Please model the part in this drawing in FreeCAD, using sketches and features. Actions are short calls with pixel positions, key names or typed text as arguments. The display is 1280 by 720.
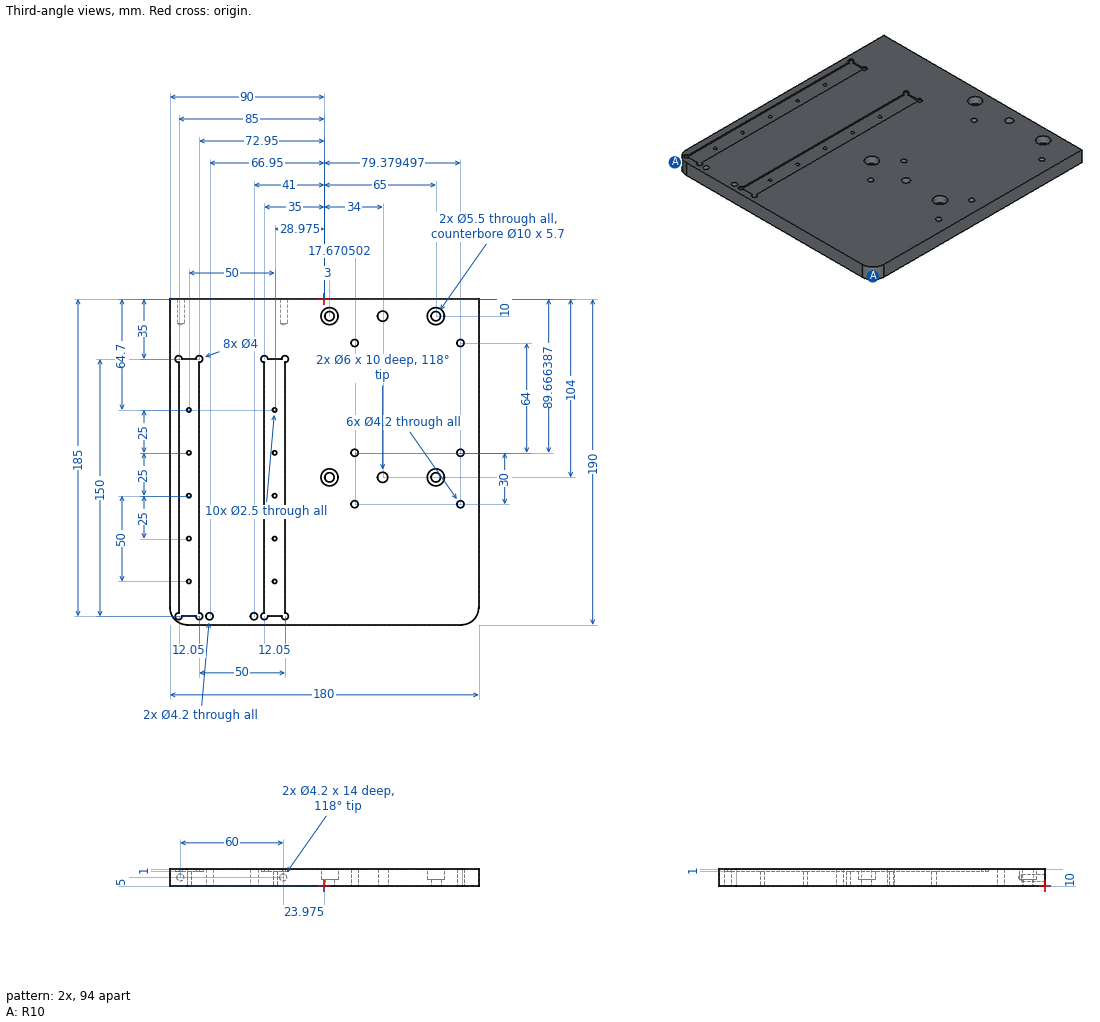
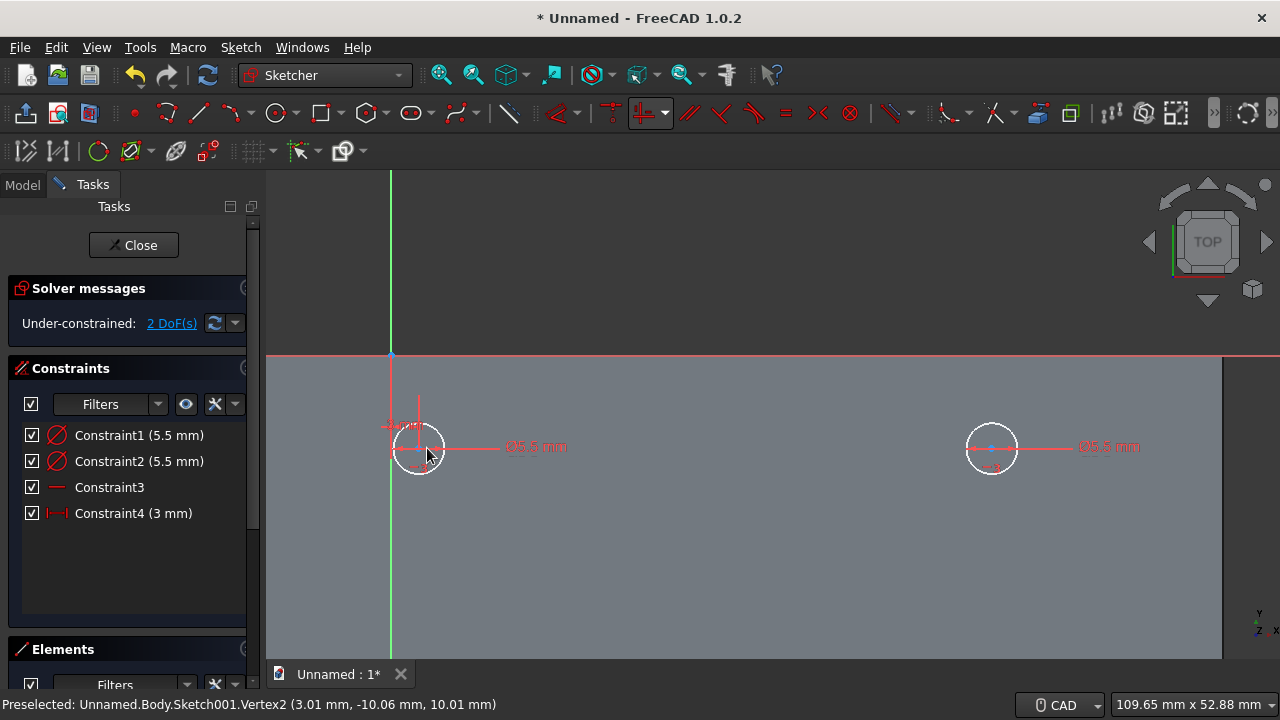
click(992, 449)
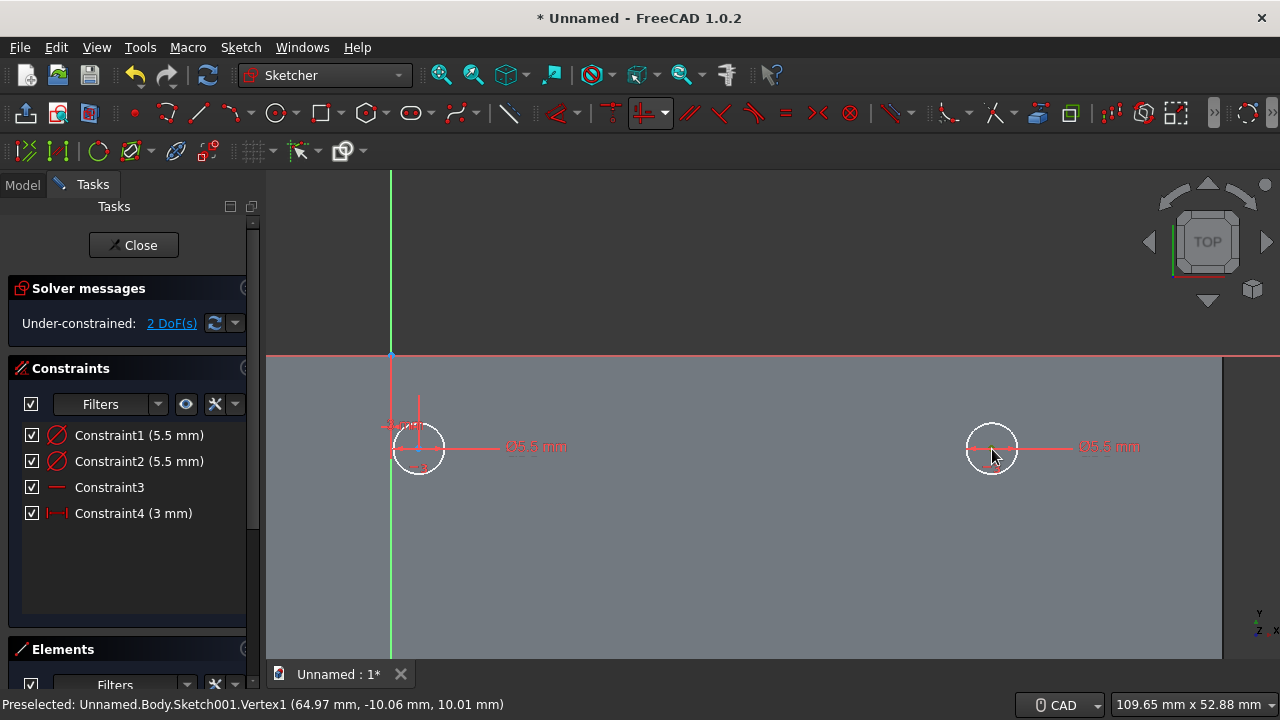
key(l)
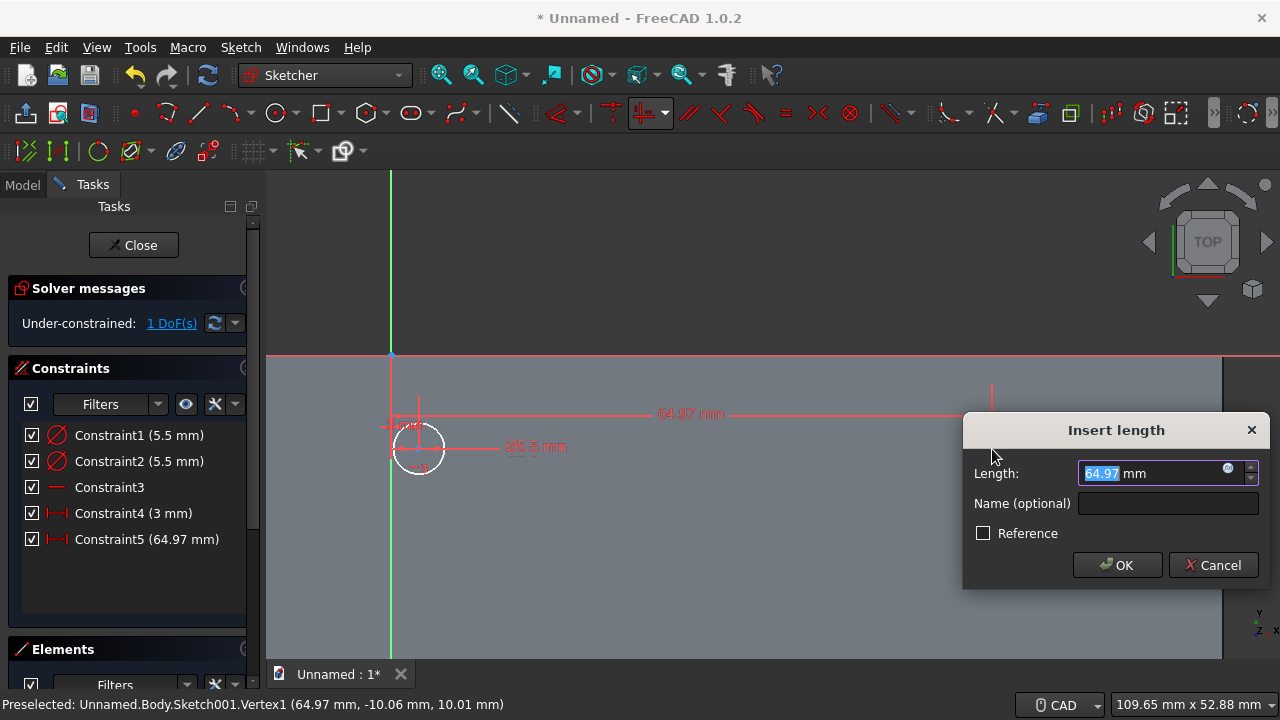
text(65)
key(Return)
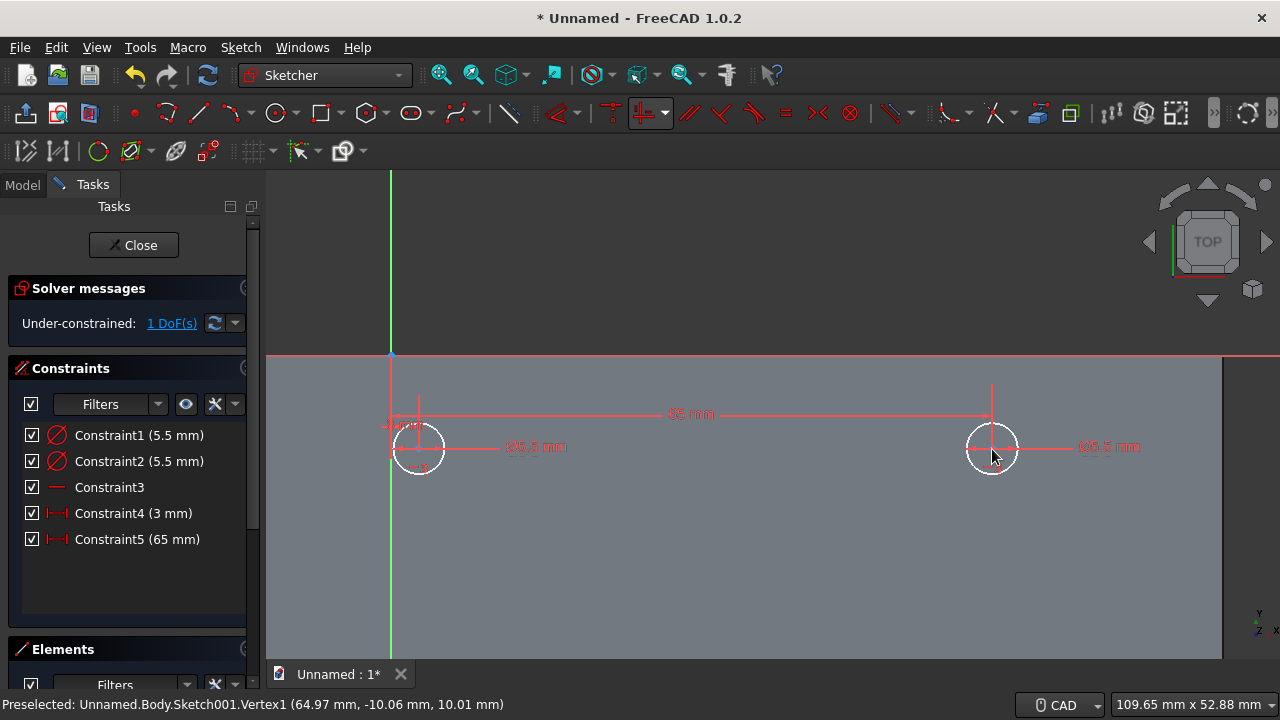
click(992, 449)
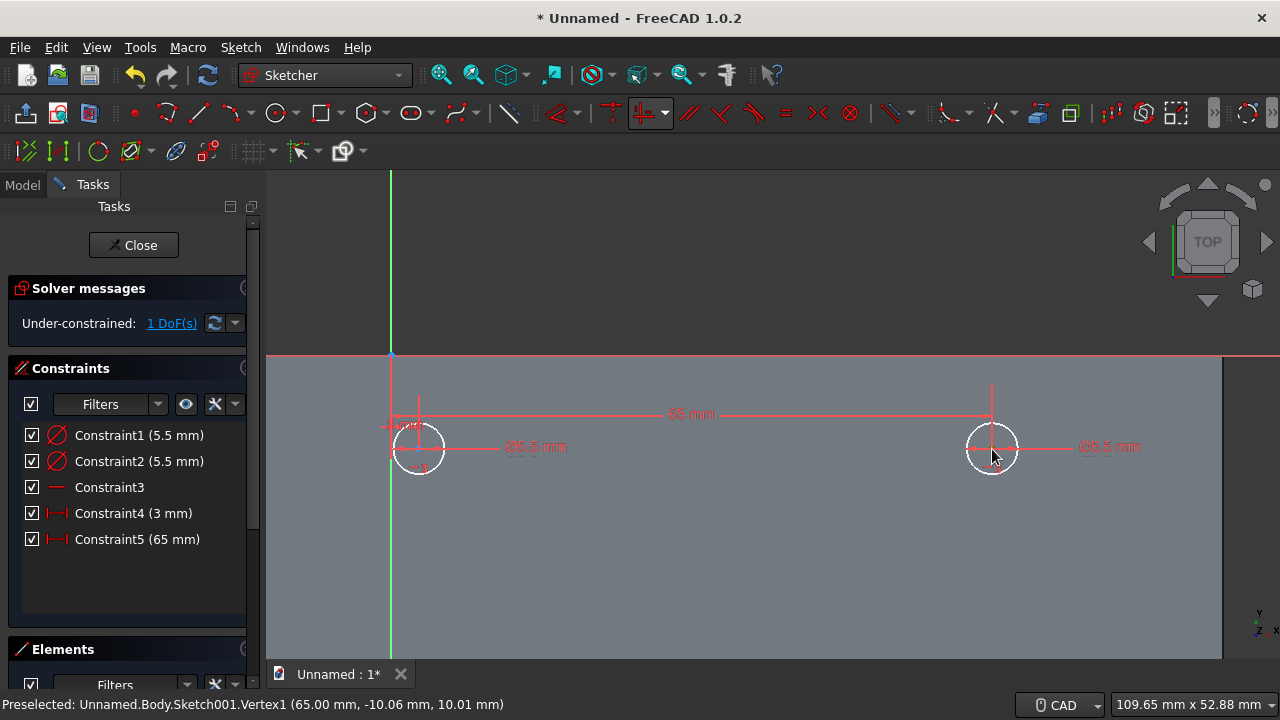
key(i)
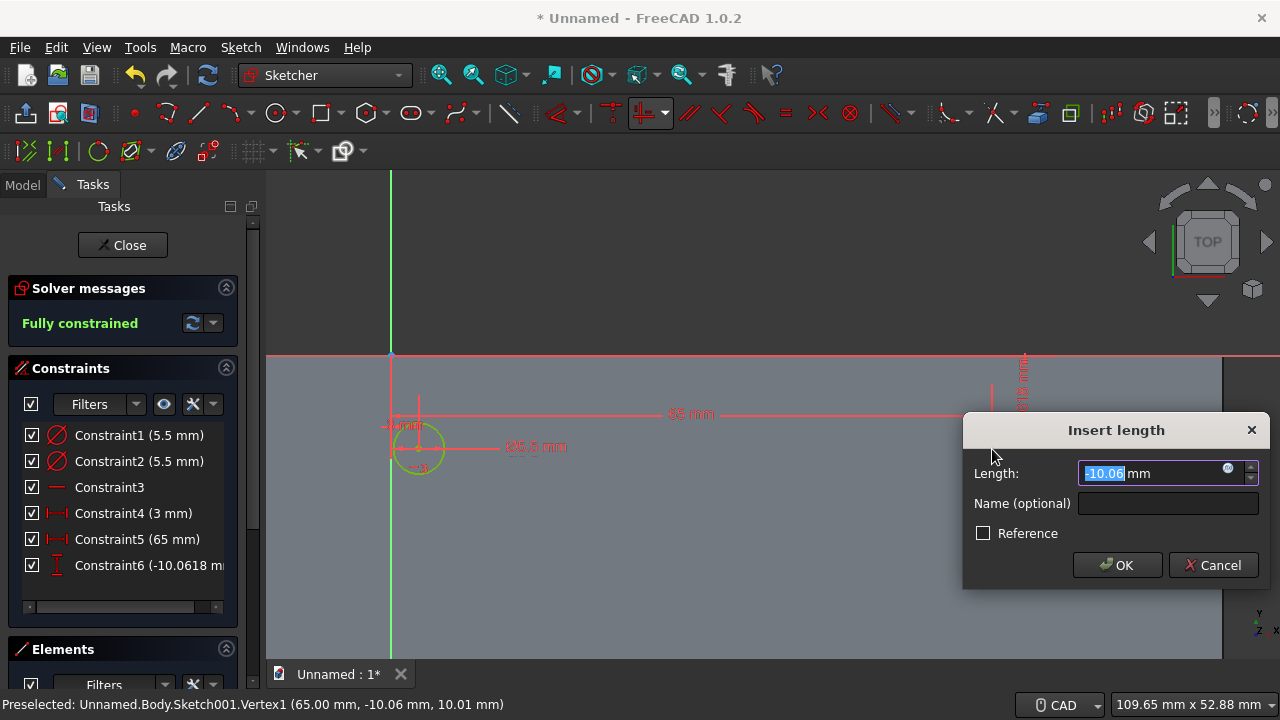
text(-10)
key(Return)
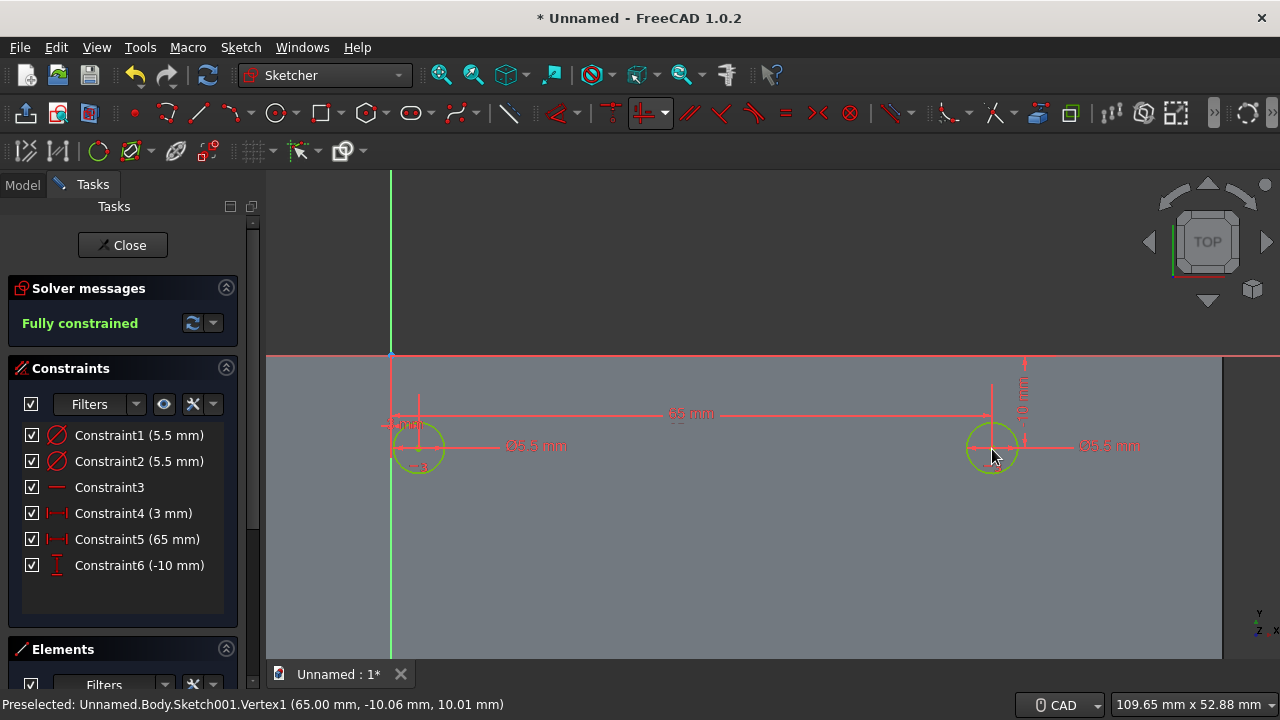
click(123, 245)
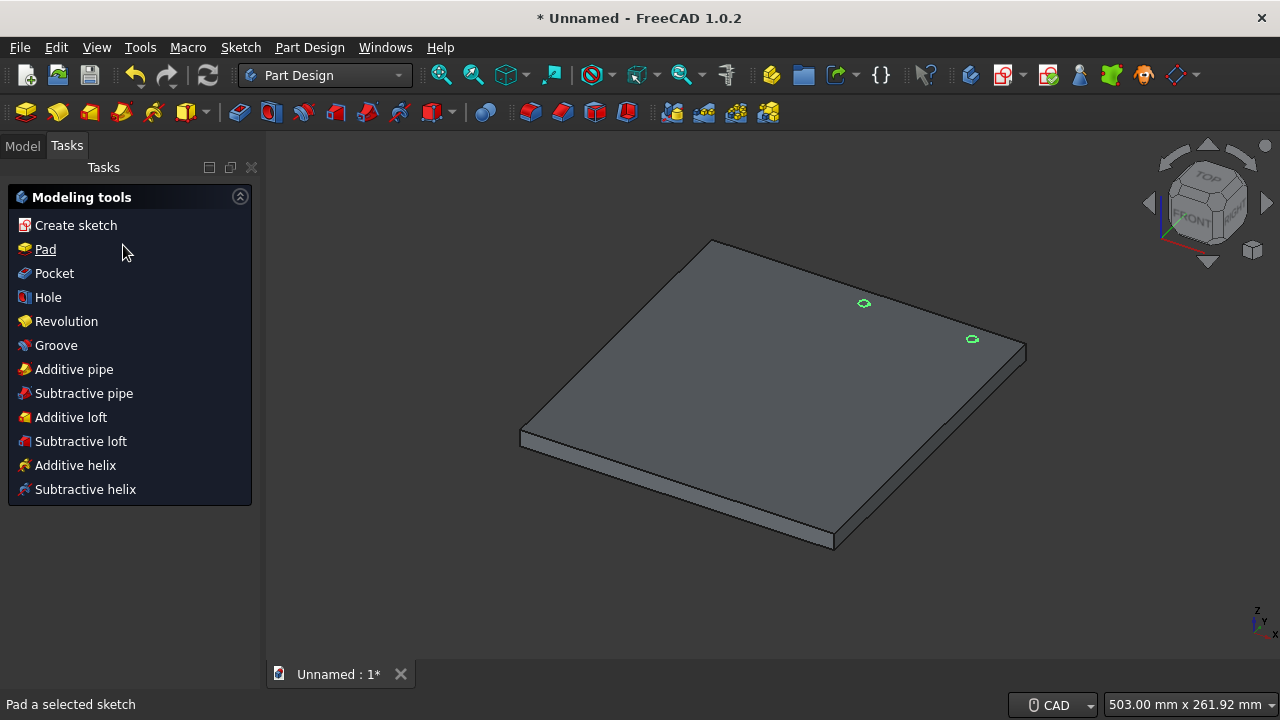
click(272, 112)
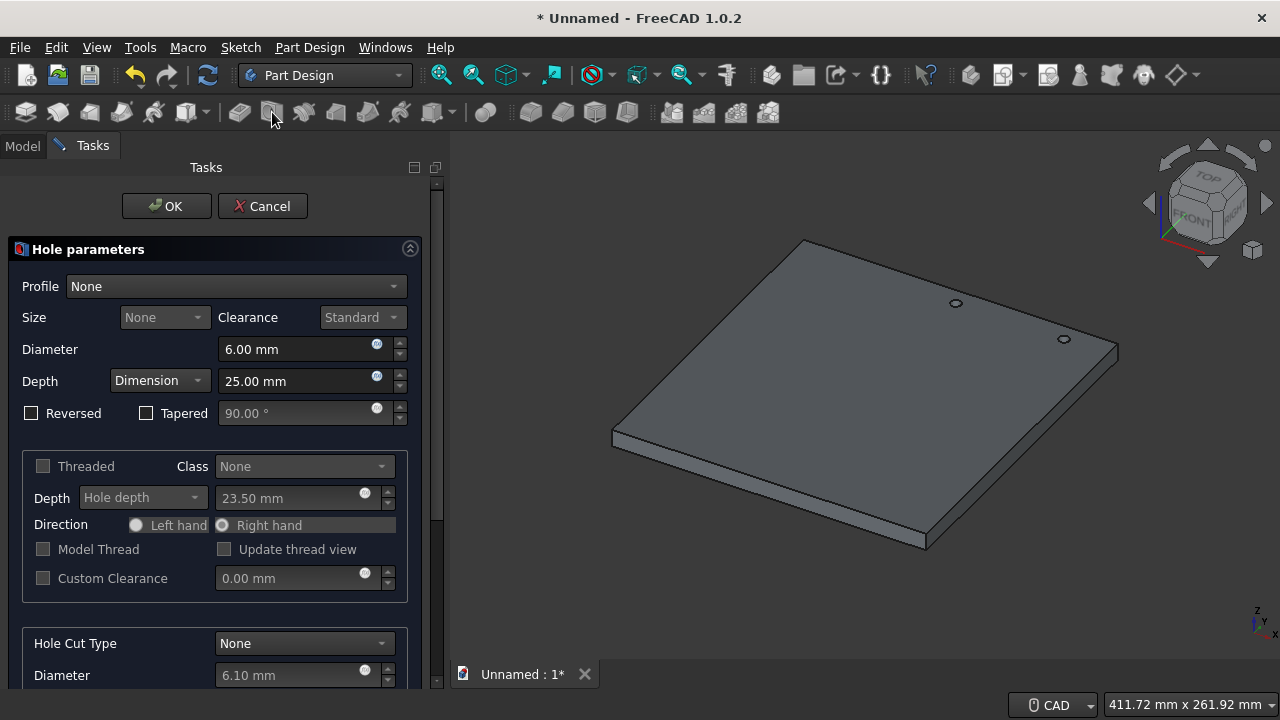
triple_click(305, 349)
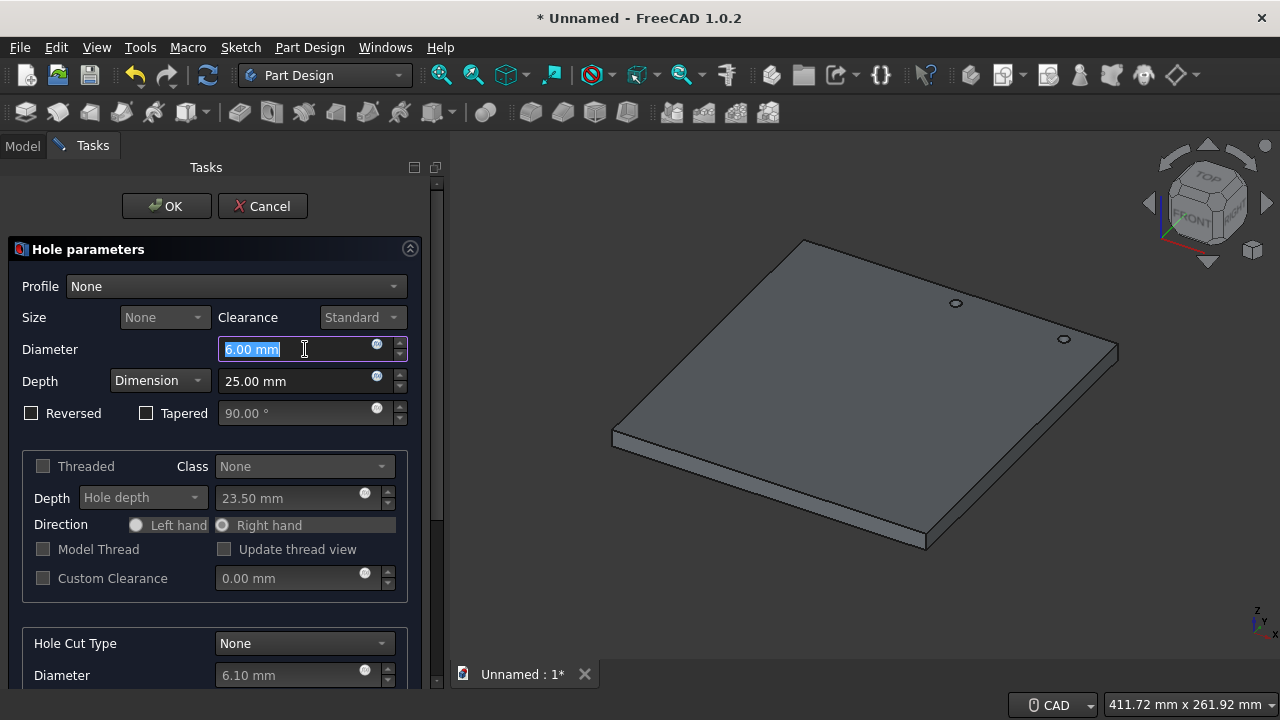
text(5.5)
key(Tab)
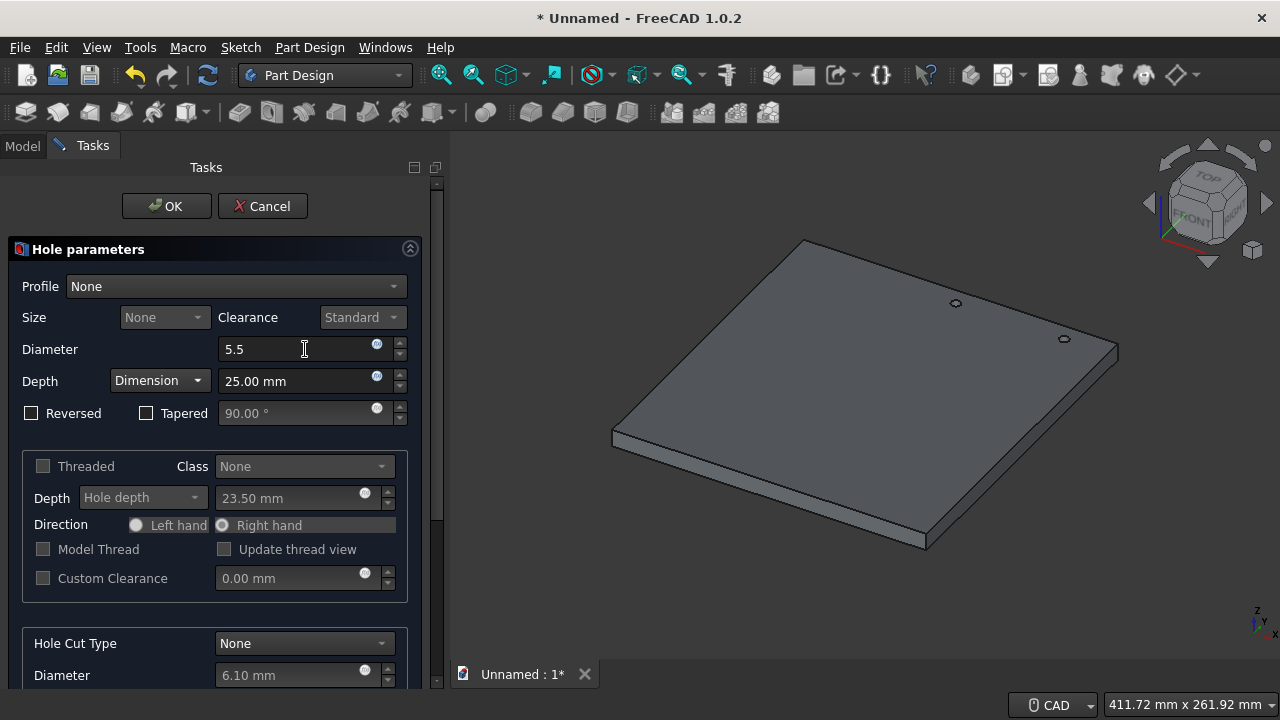
click(161, 380)